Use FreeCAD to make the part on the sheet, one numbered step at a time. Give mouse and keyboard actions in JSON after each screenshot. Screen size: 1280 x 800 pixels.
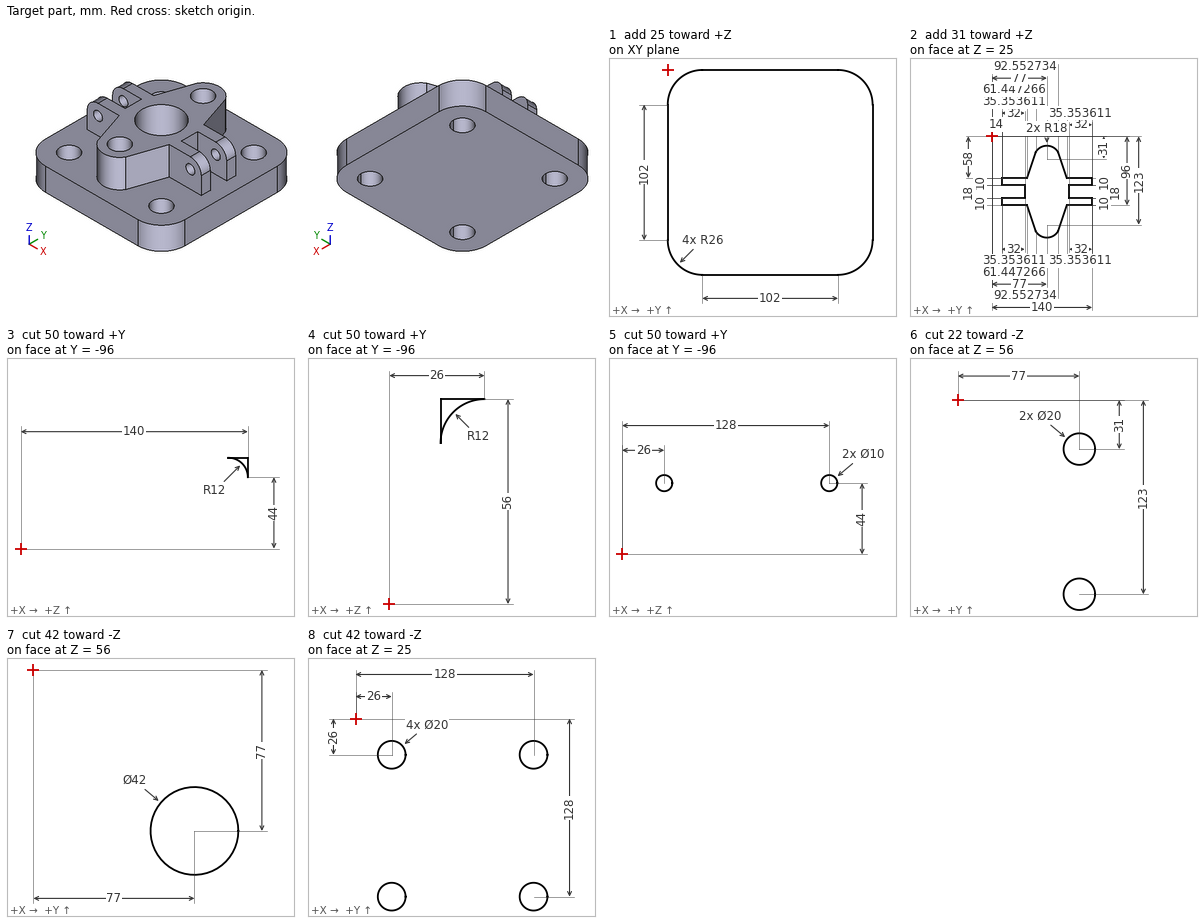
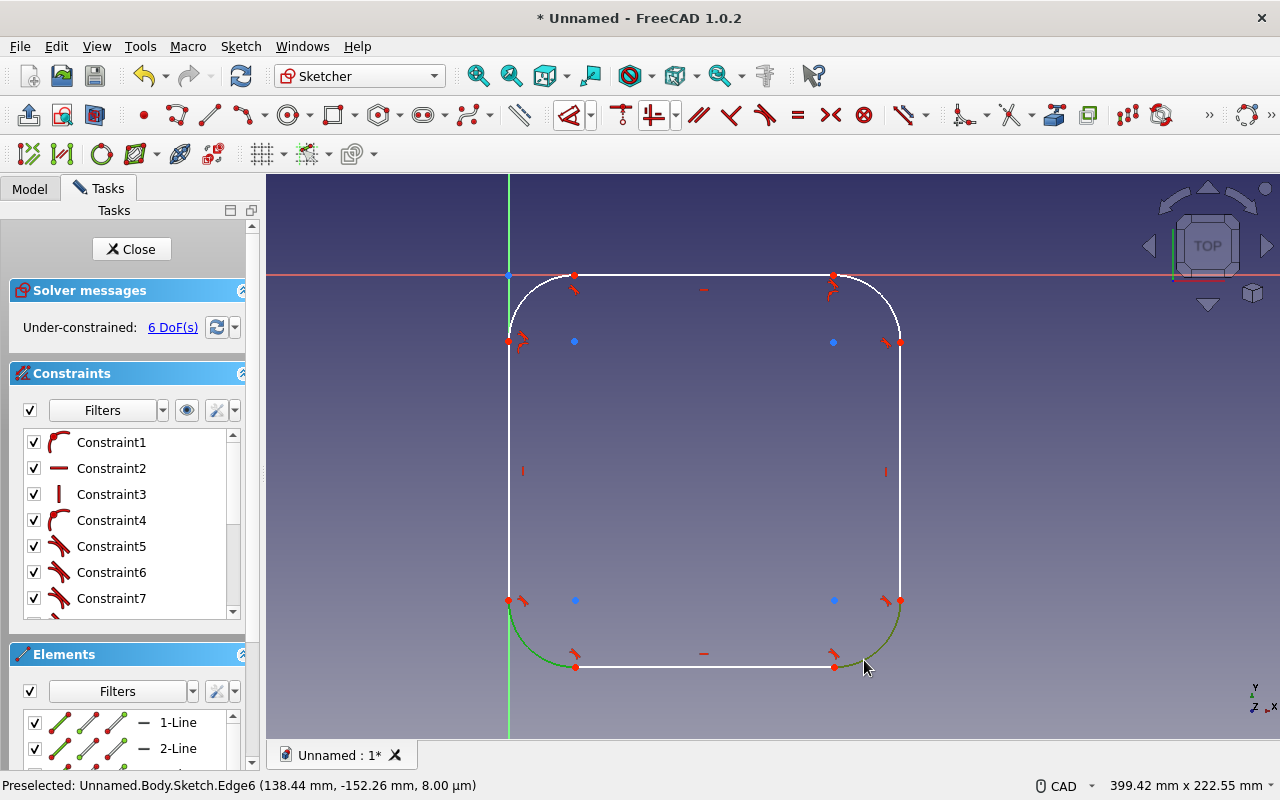
{"action": "left_click", "coordinate": [893, 312]}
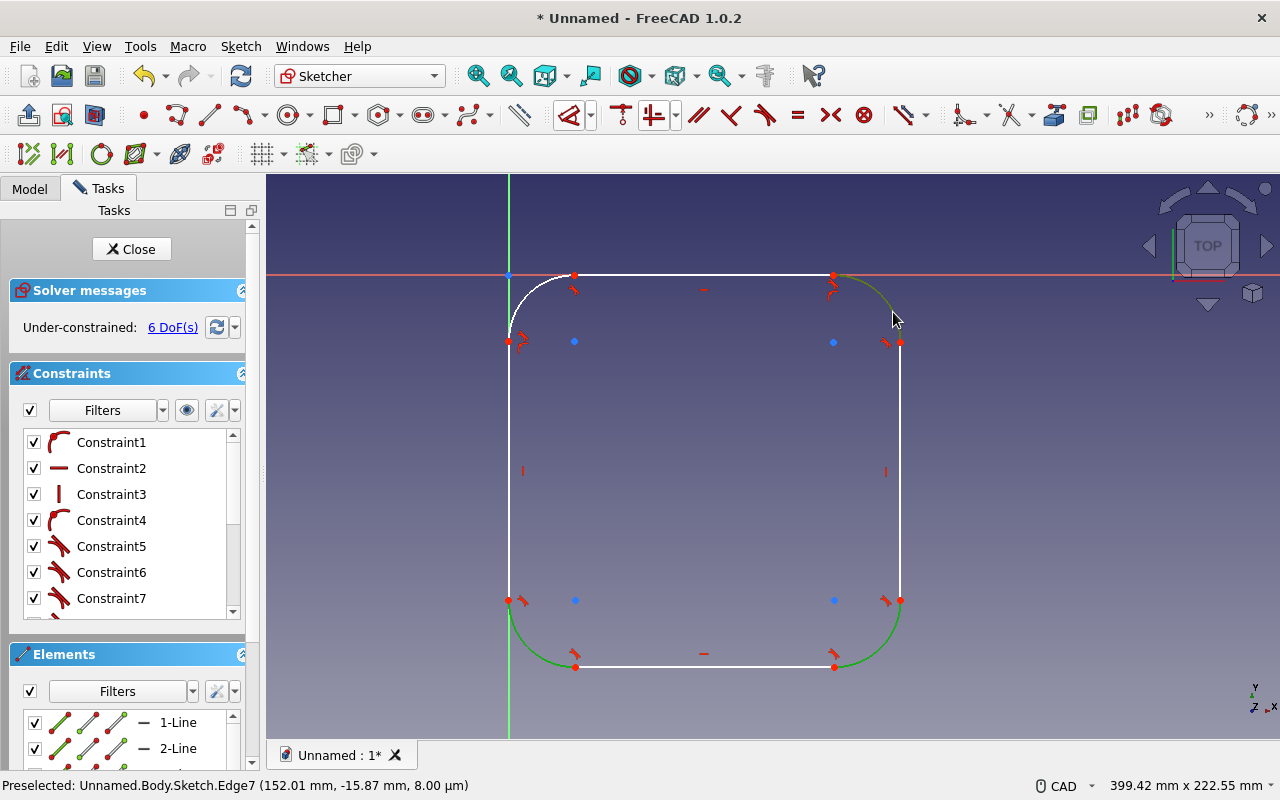
{"action": "left_click", "coordinate": [528, 294]}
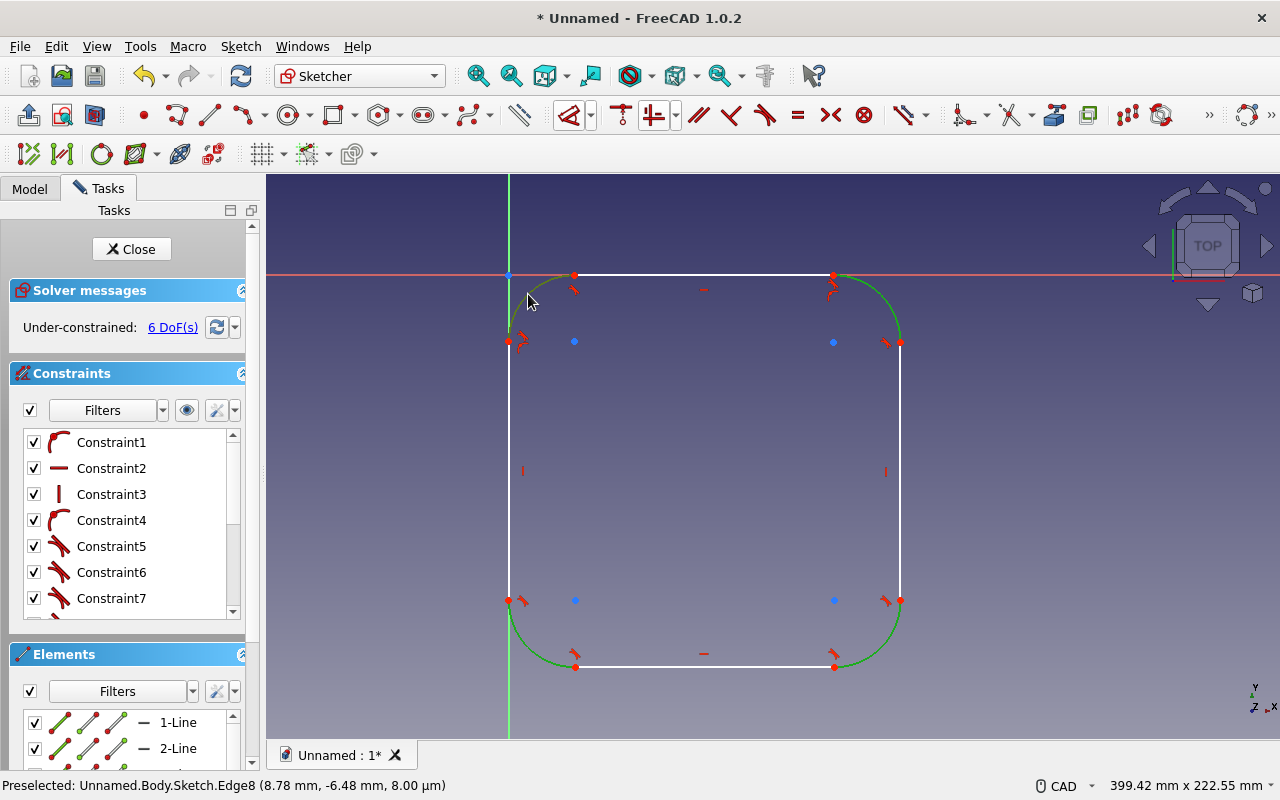
{"action": "left_click", "coordinate": [798, 116]}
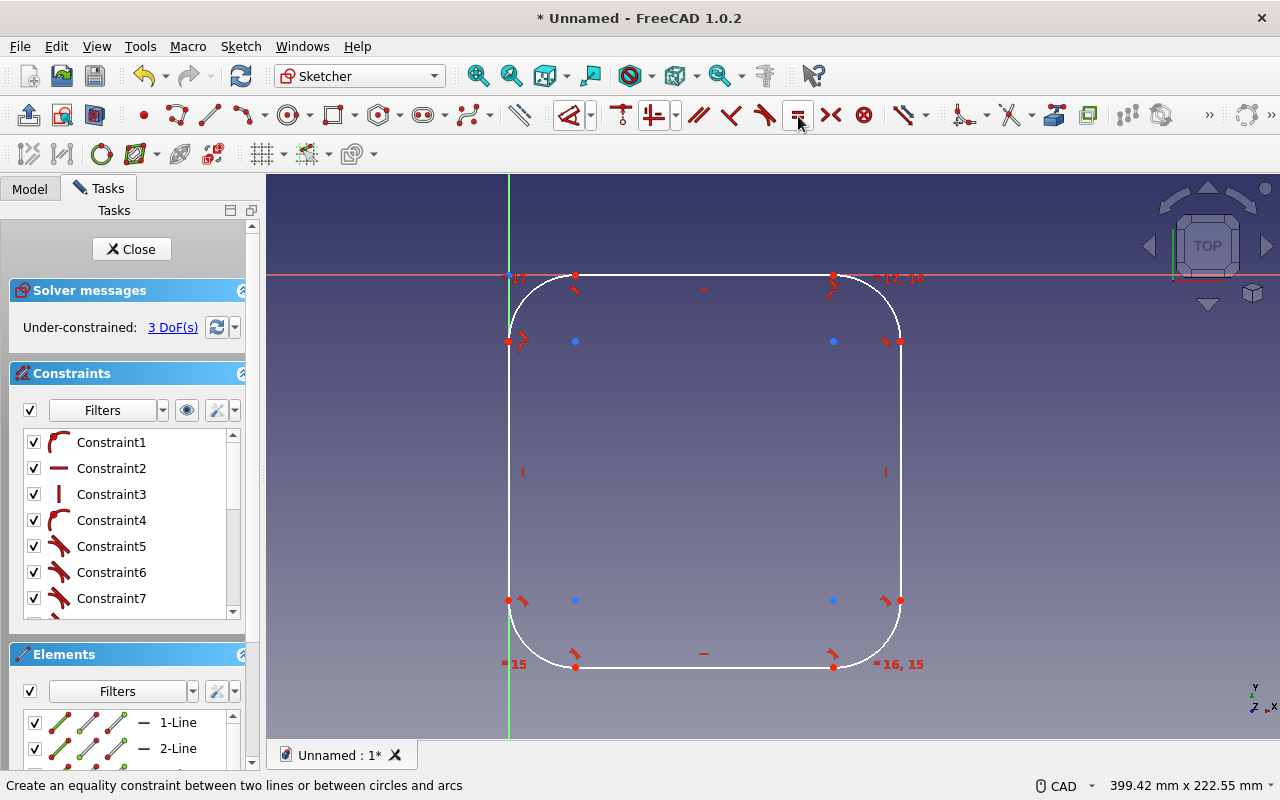
{"action": "left_click", "coordinate": [545, 660]}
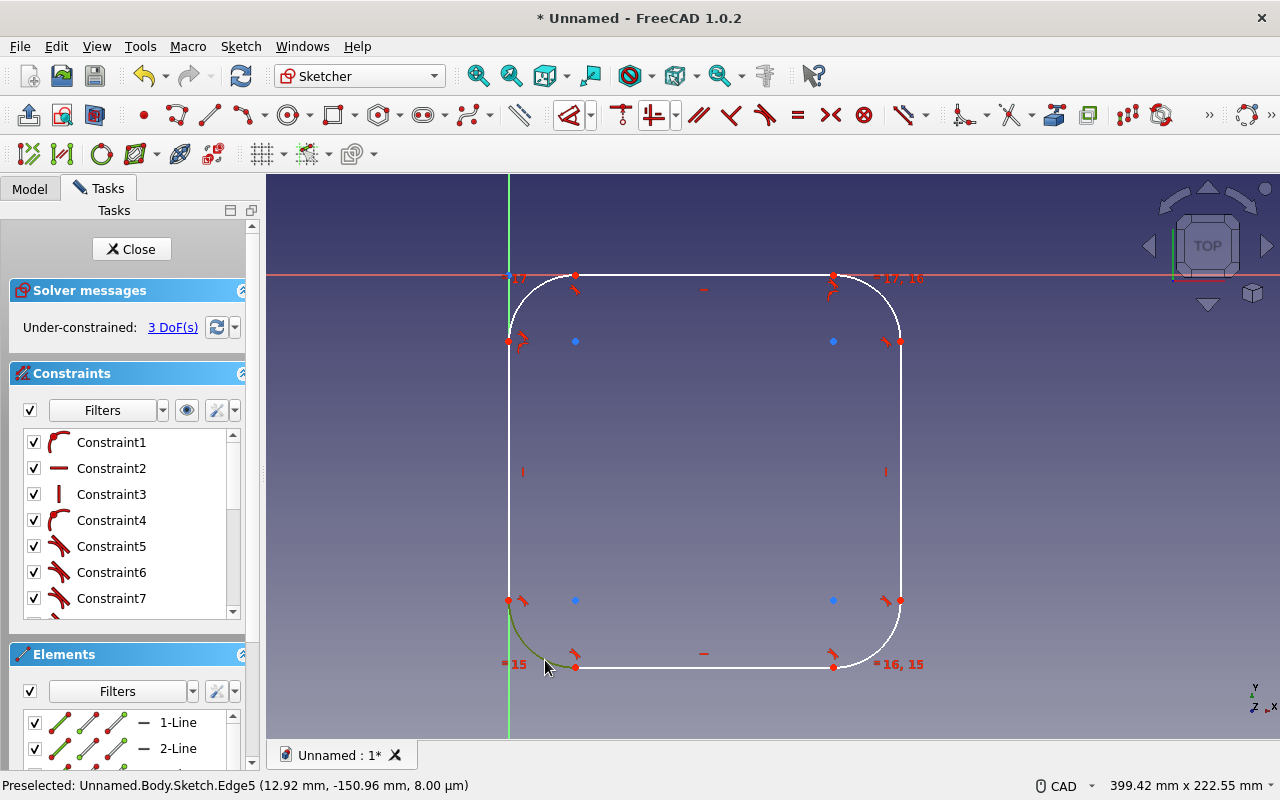
{"action": "key", "text": "k r"}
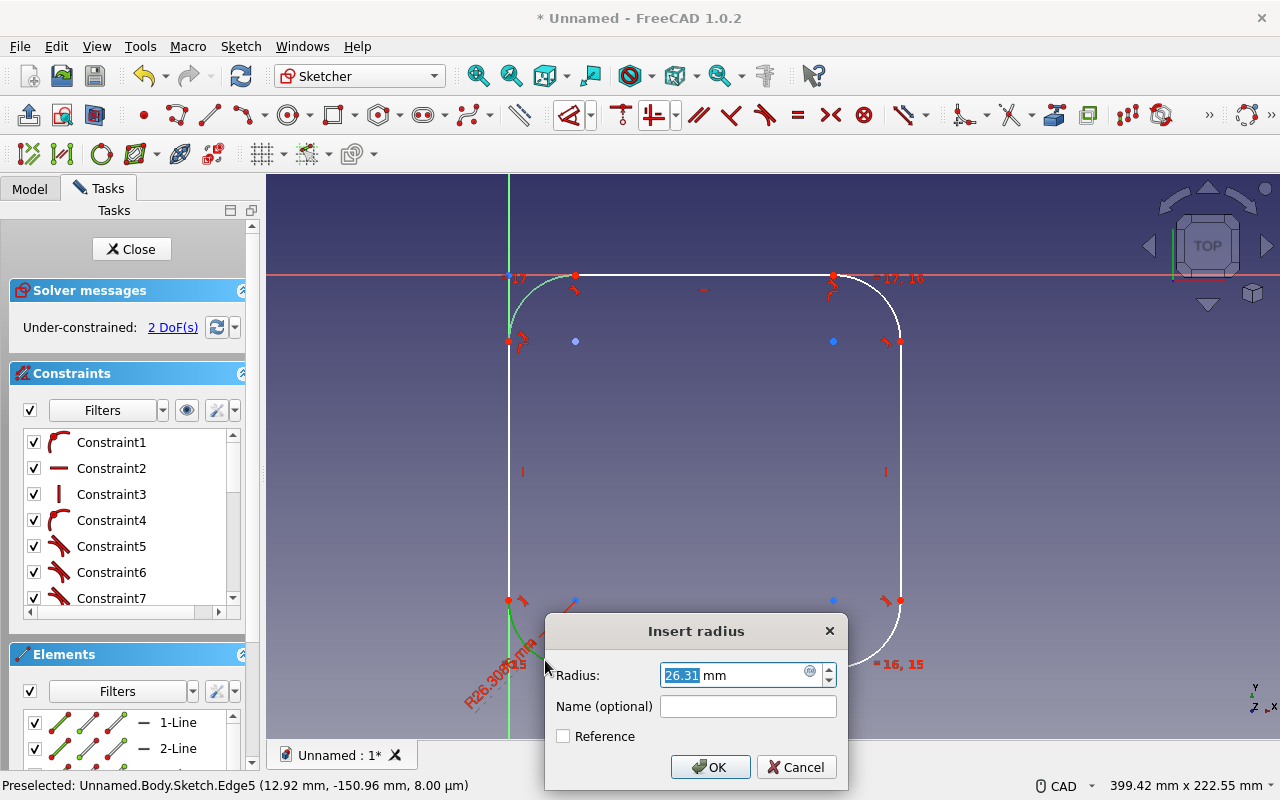
{"action": "type", "text": "26"}
{"action": "key", "text": "Return"}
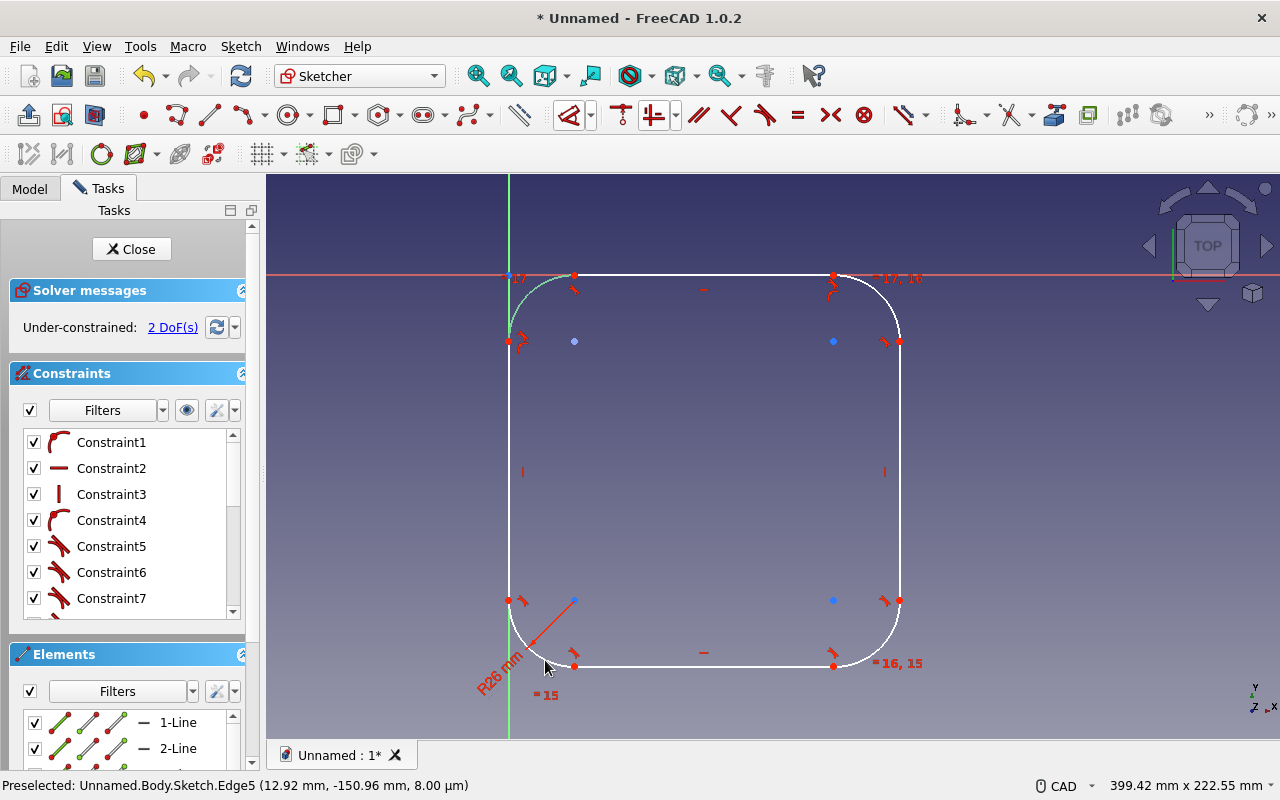
{"action": "left_click", "coordinate": [509, 419]}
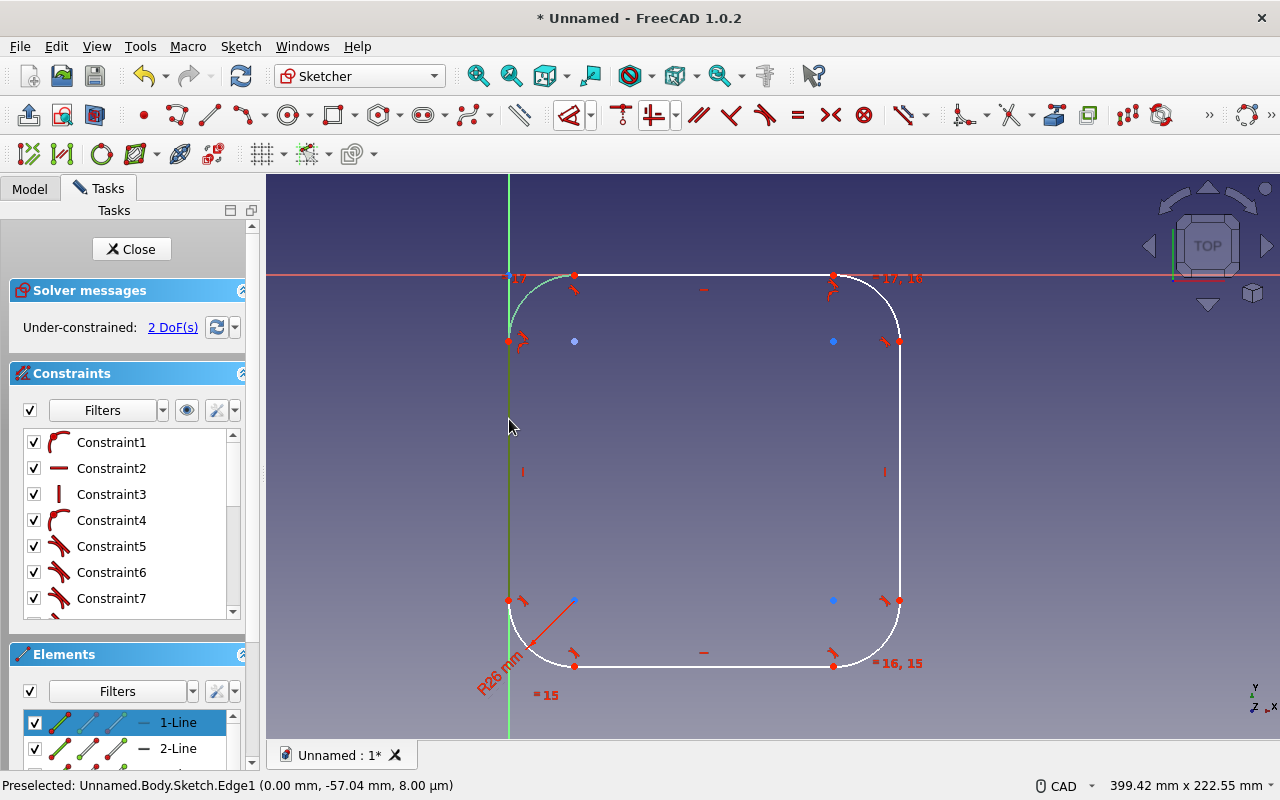
{"action": "left_click", "coordinate": [590, 116]}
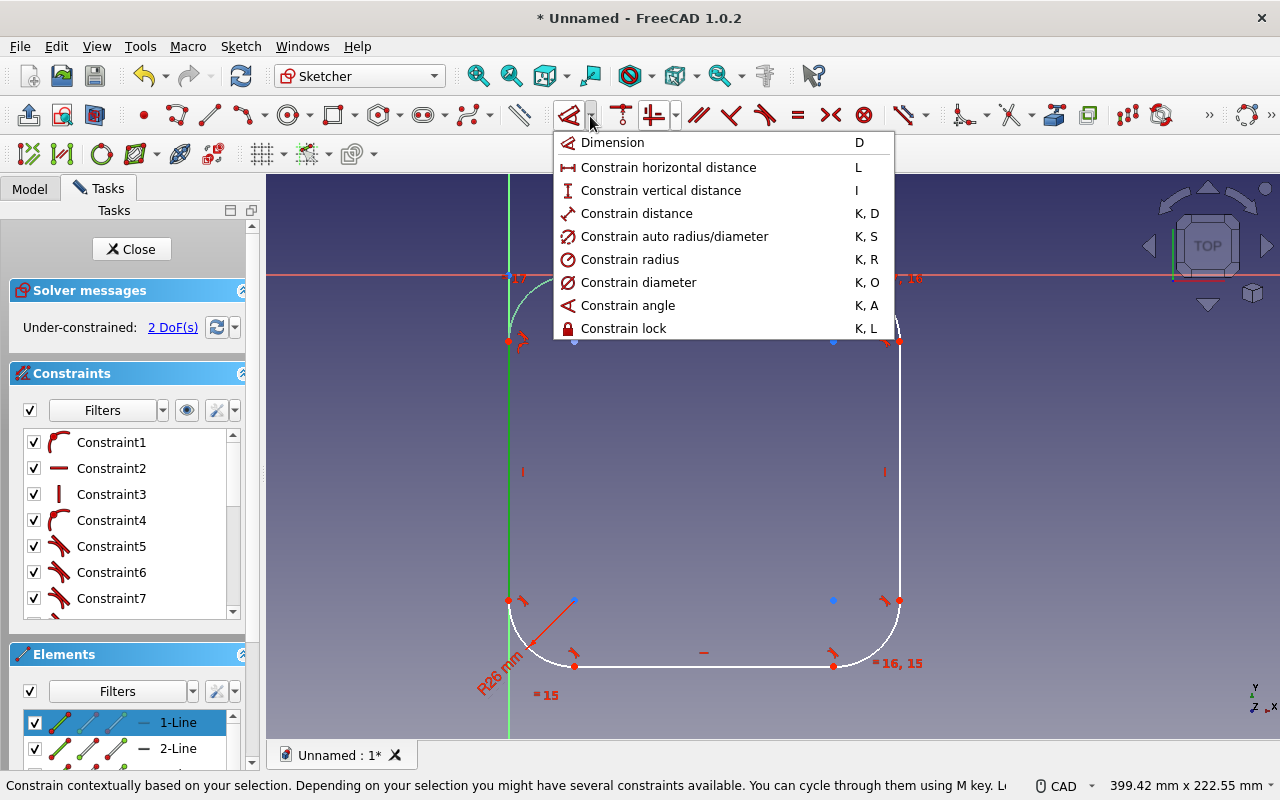
{"action": "left_click", "coordinate": [724, 190]}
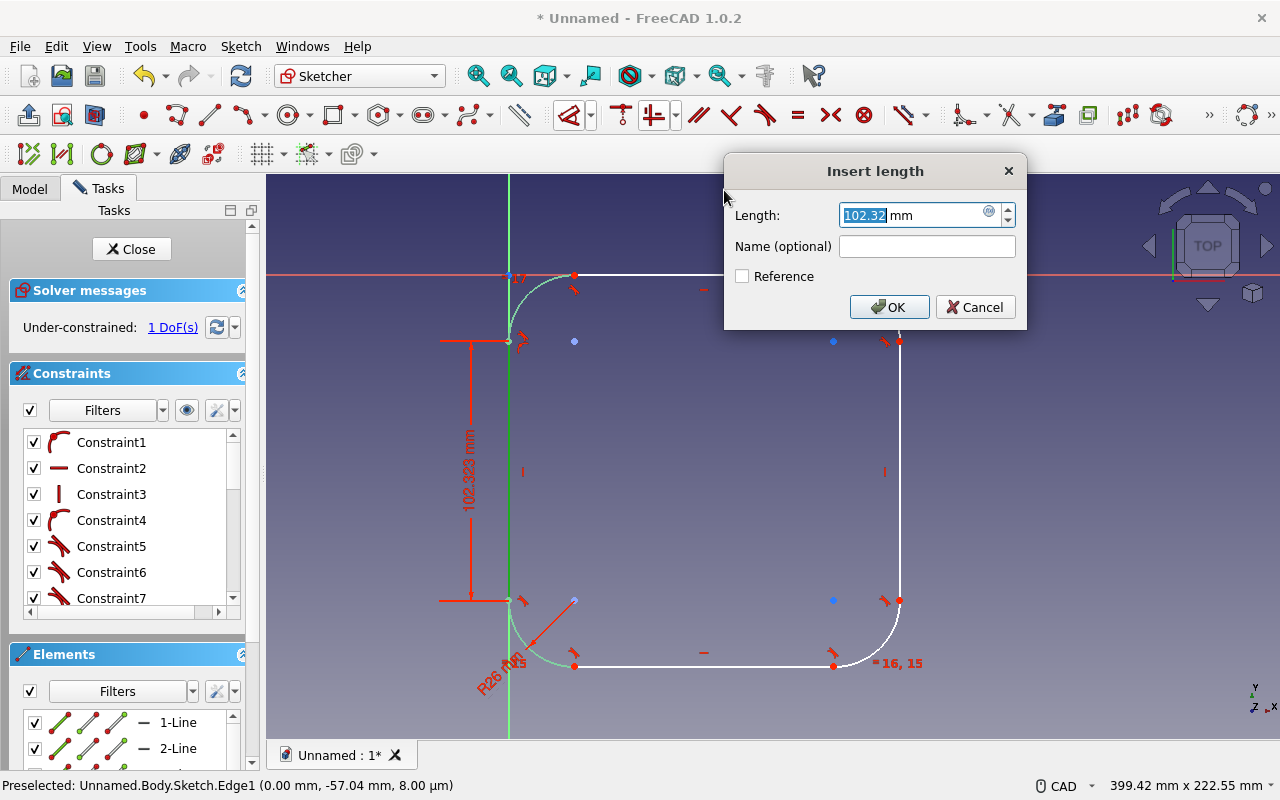
{"action": "type", "text": "102"}
{"action": "key", "text": "Return"}